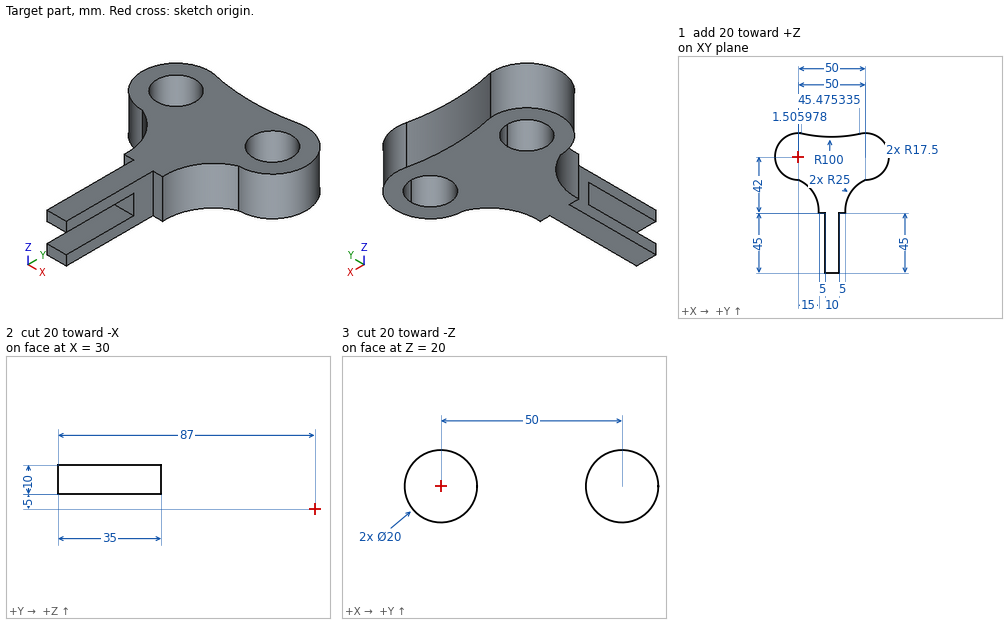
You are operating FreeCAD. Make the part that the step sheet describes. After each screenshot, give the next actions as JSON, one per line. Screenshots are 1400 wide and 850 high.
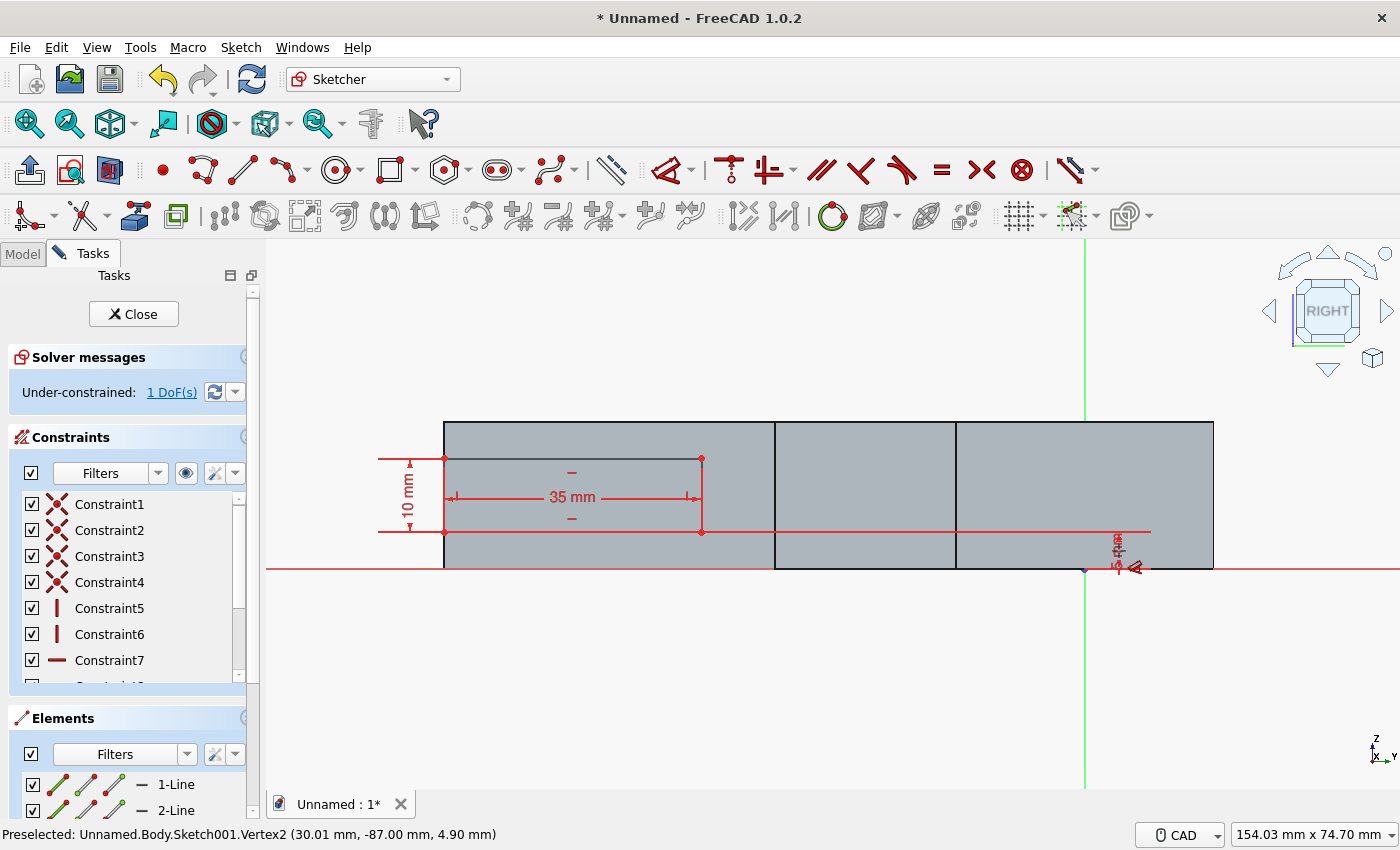
{"action": "left_click", "coordinate": [444, 459]}
{"action": "left_click", "coordinate": [764, 603]}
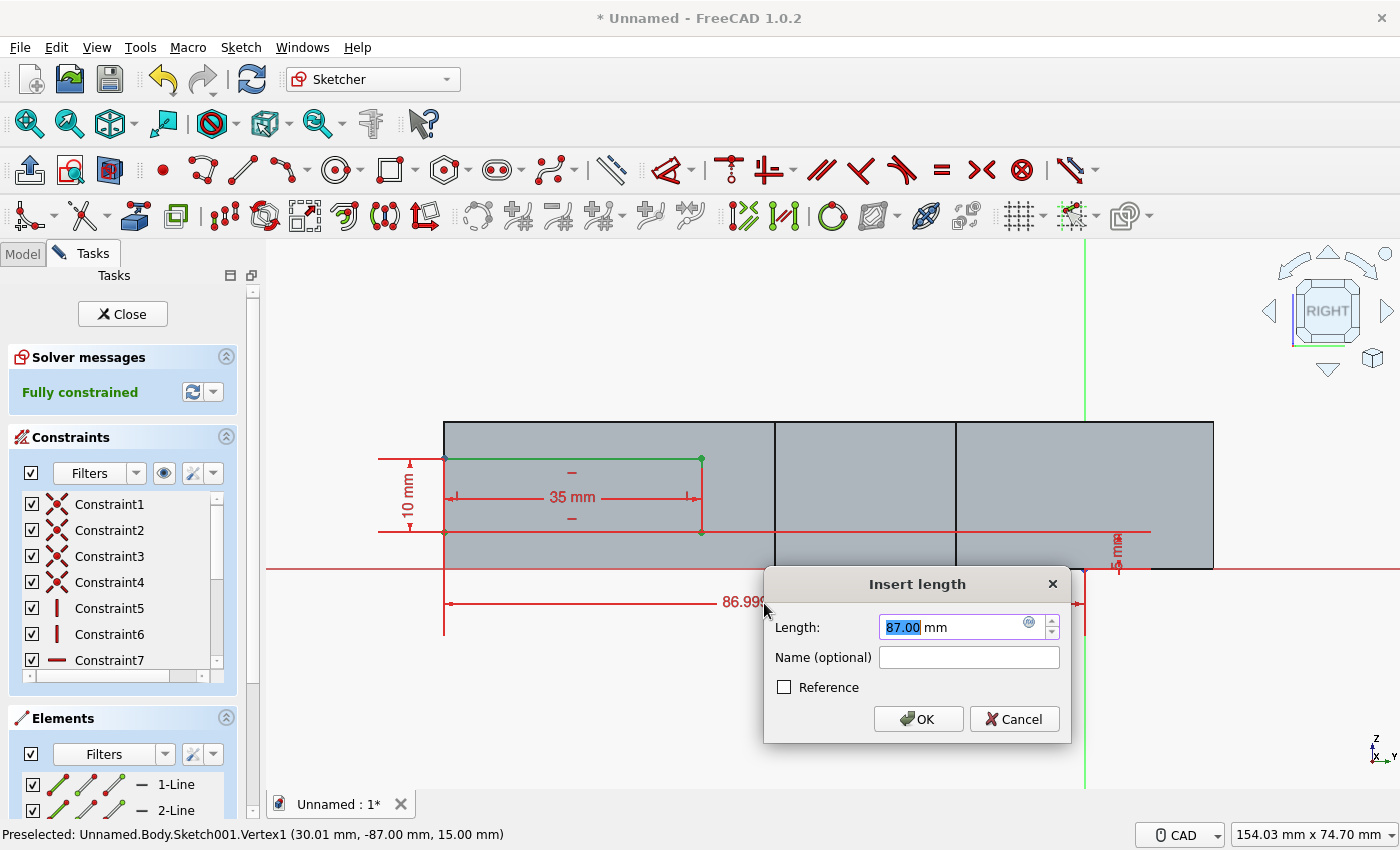
{"action": "type", "text": "87"}
{"action": "key", "text": "Return"}
{"action": "key", "text": "Escape"}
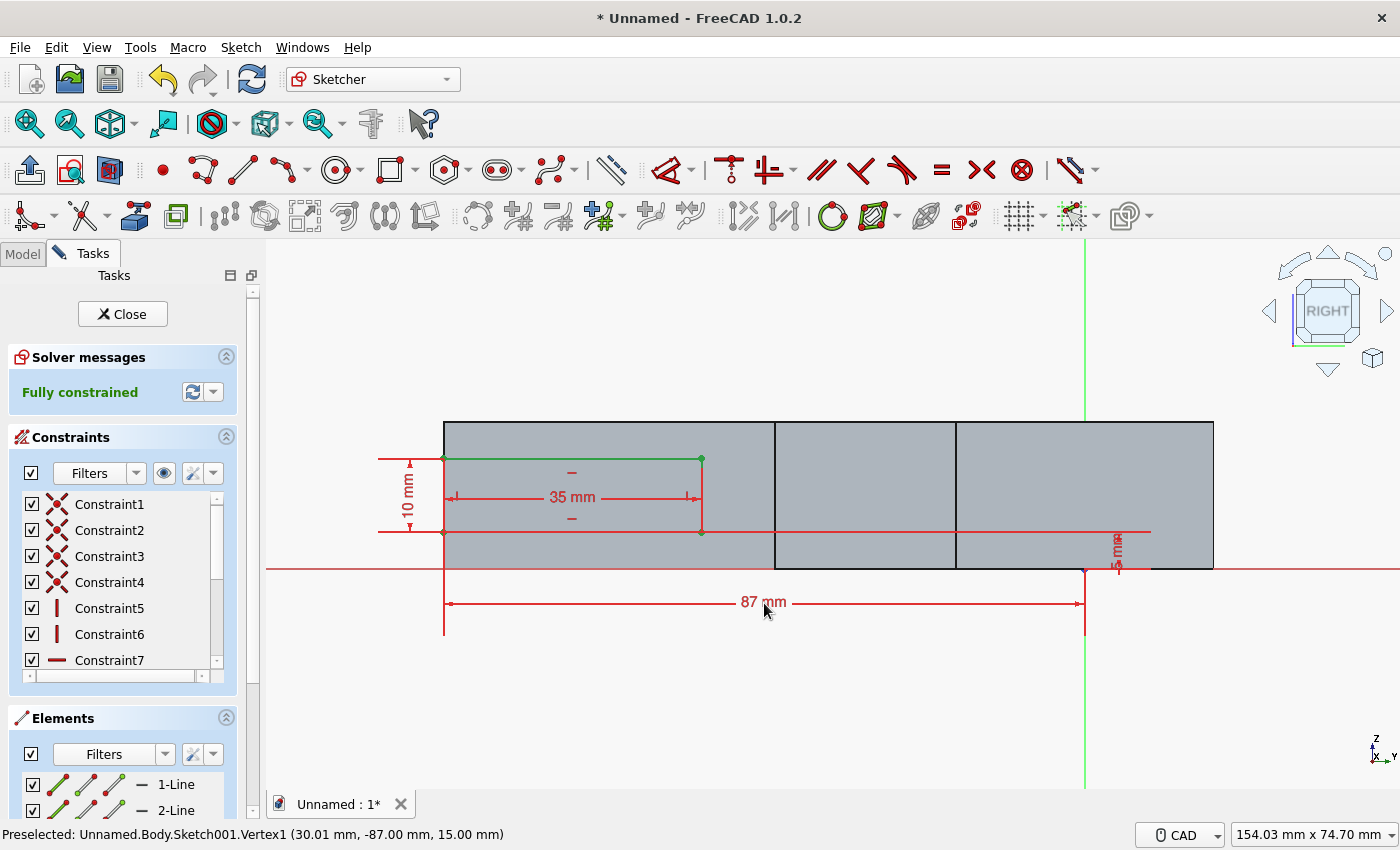
{"action": "left_click", "coordinate": [123, 314]}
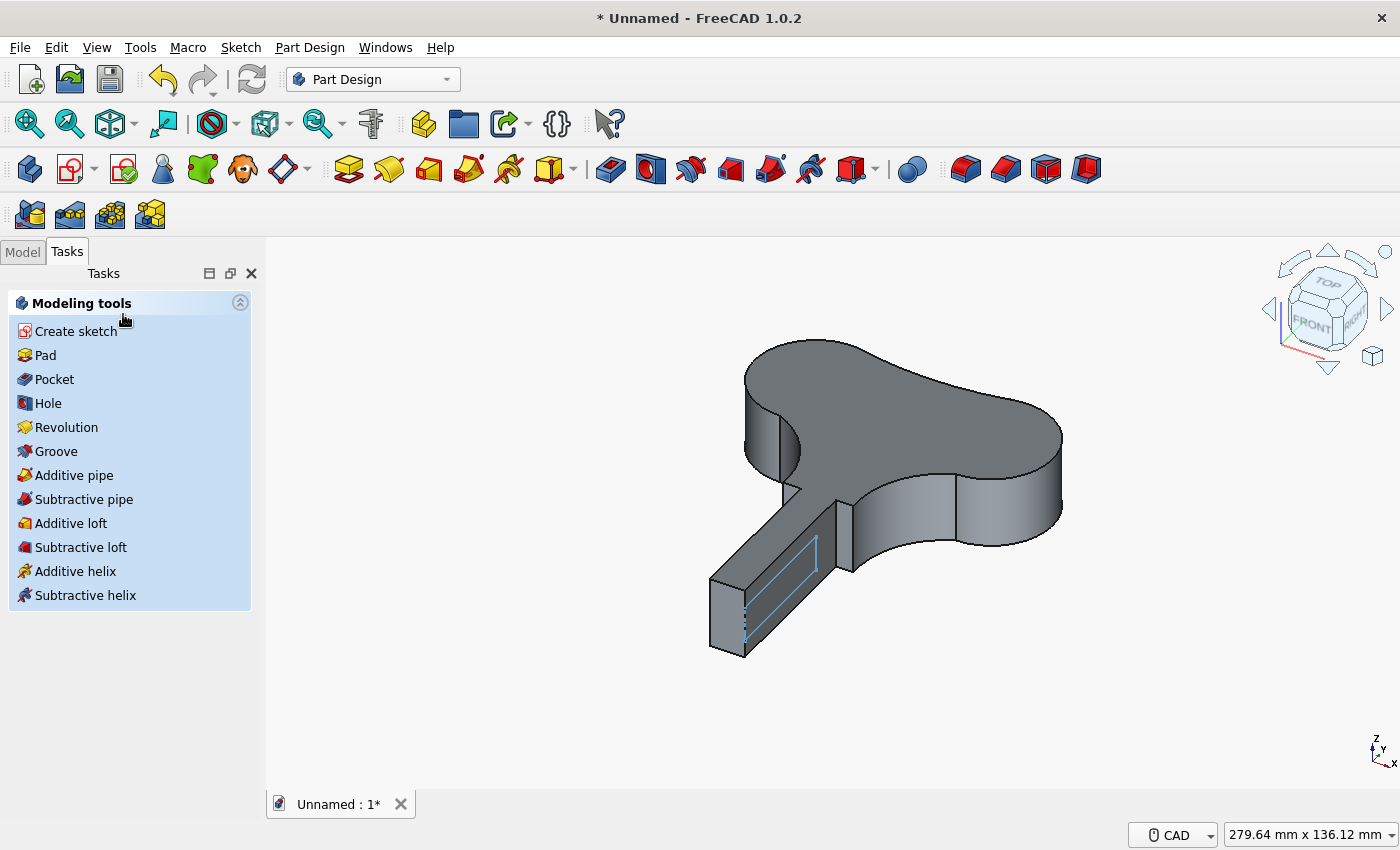
{"action": "left_click", "coordinate": [612, 170]}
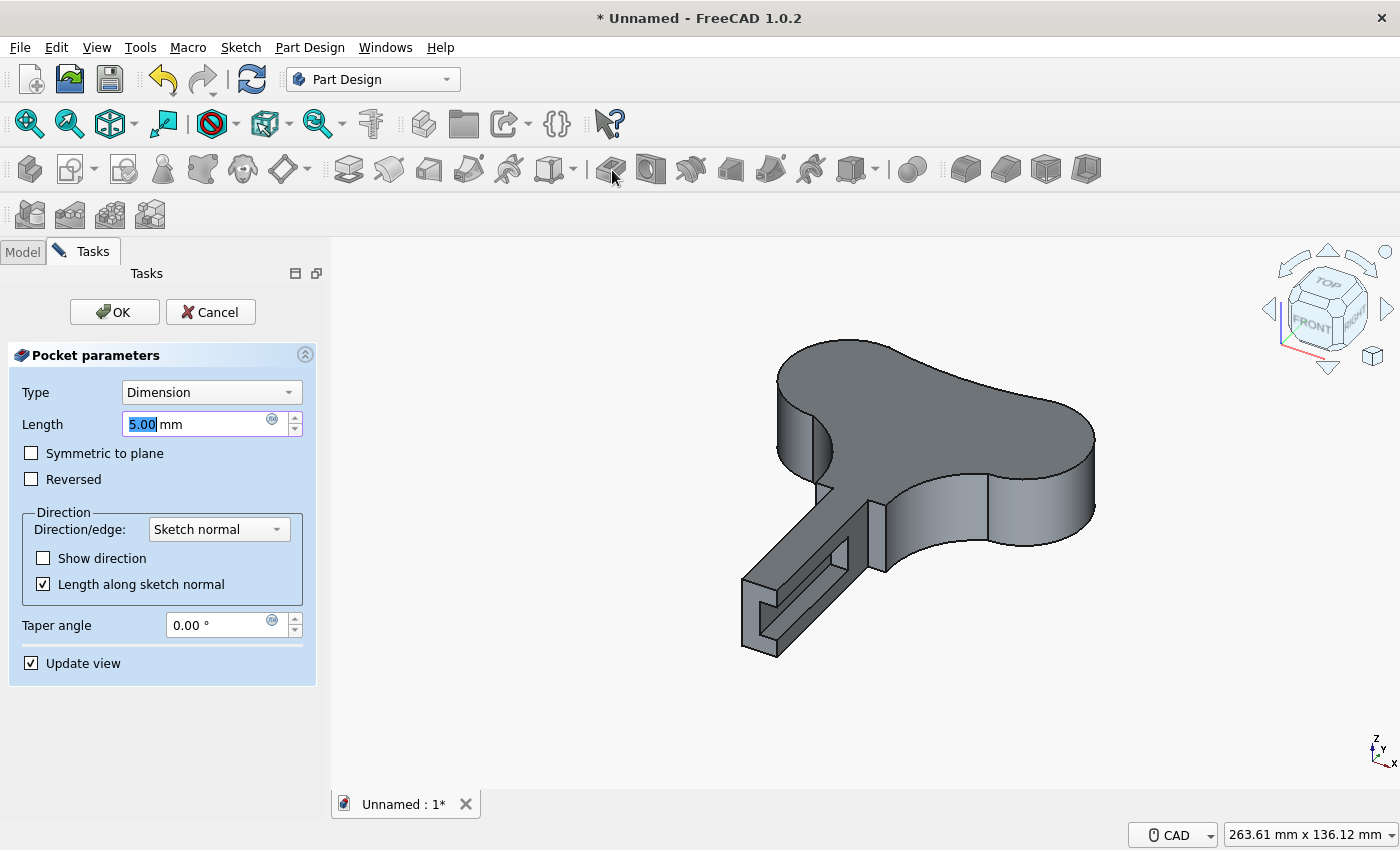
{"action": "type", "text": "20"}
{"action": "key", "text": "Tab"}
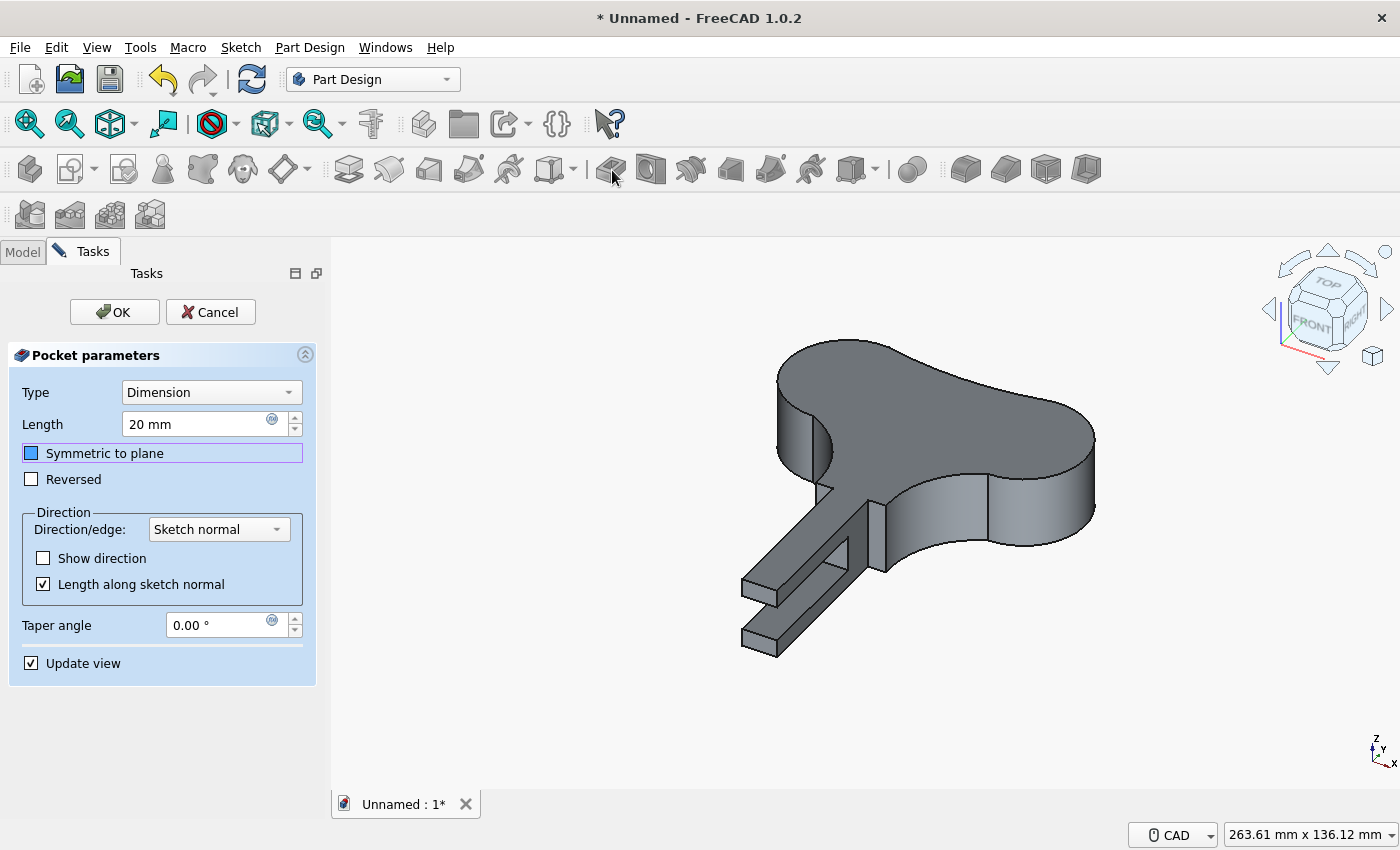
{"action": "left_click", "coordinate": [115, 312]}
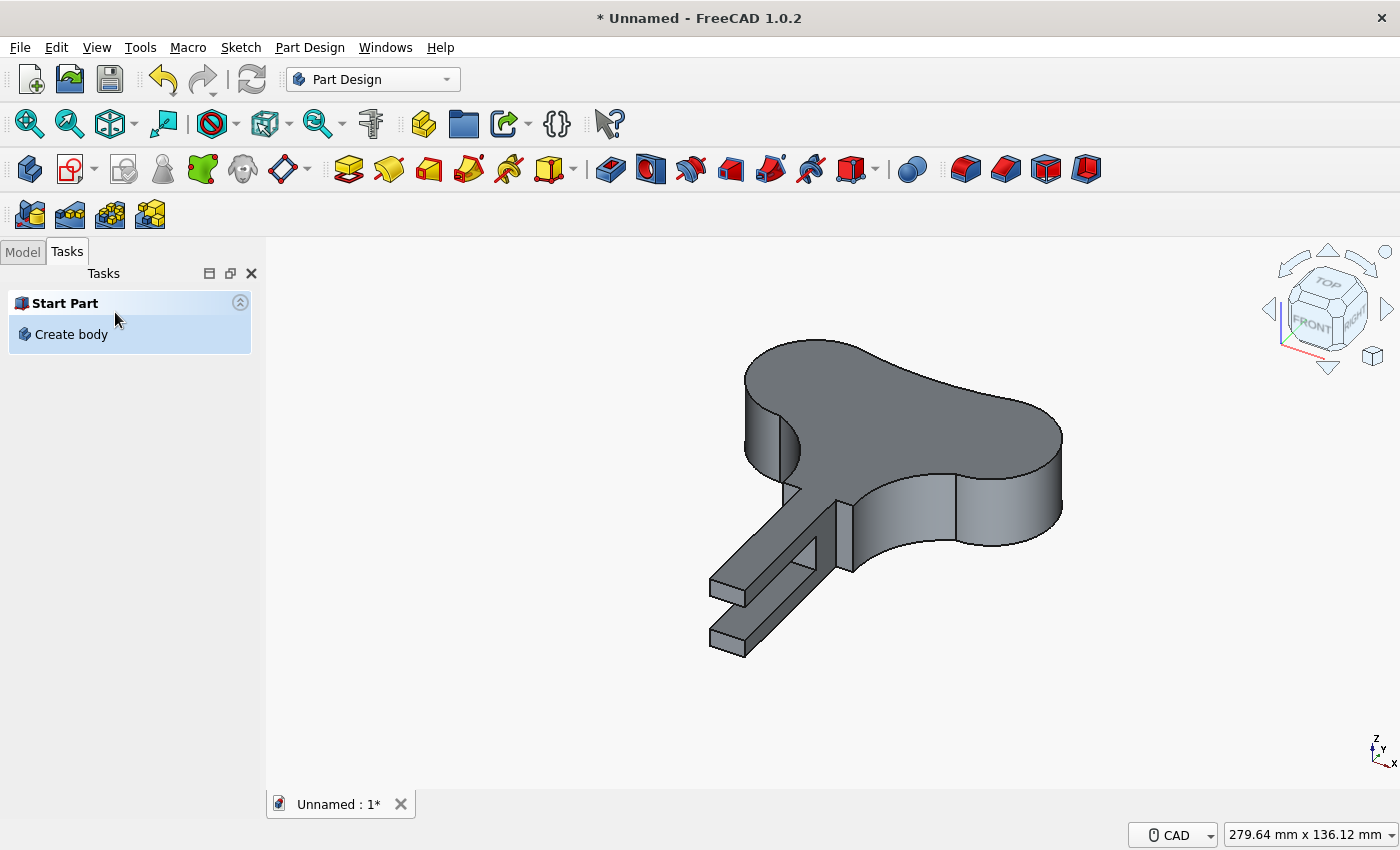
{"action": "left_click", "coordinate": [894, 419]}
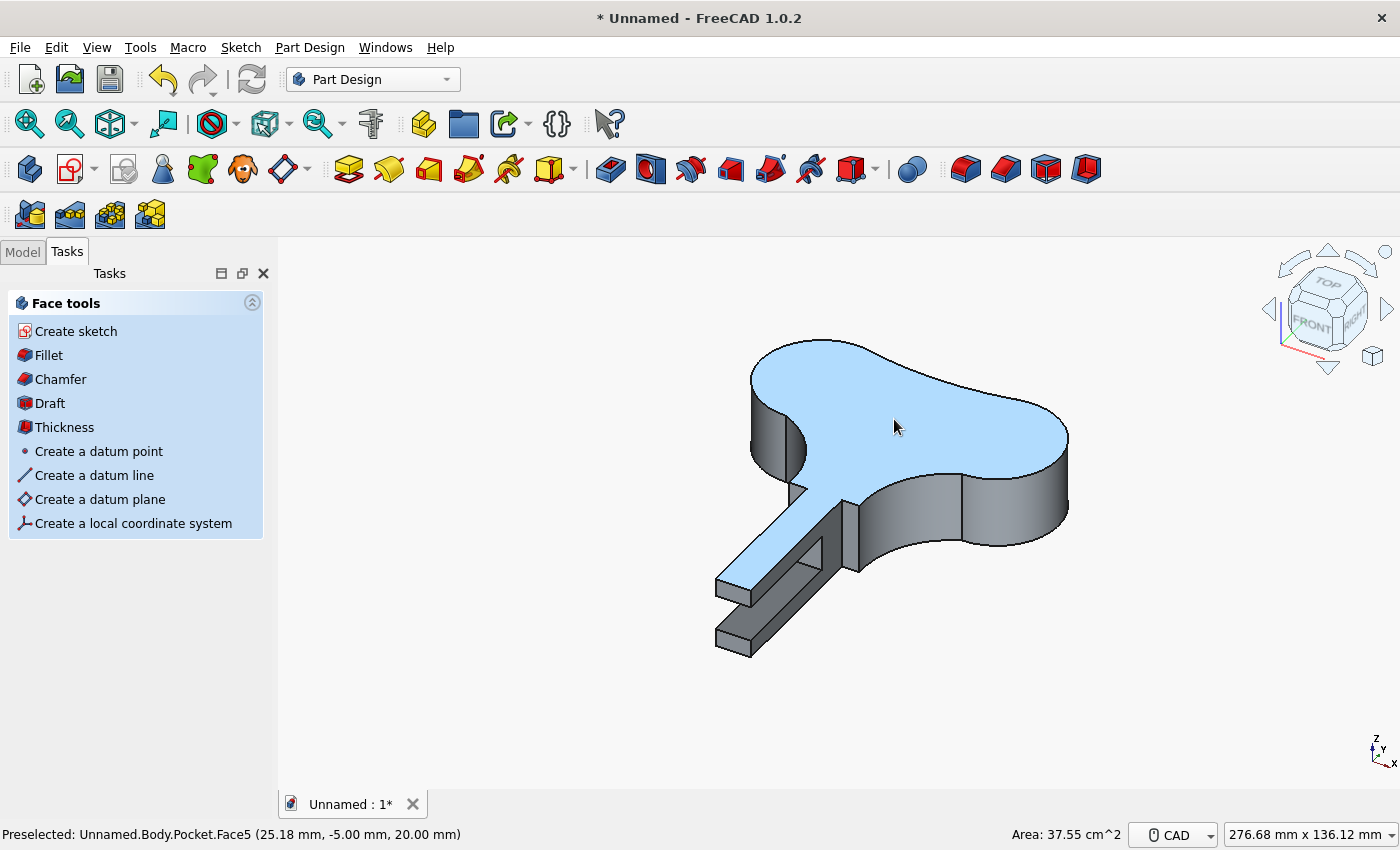
{"action": "left_click", "coordinate": [70, 170]}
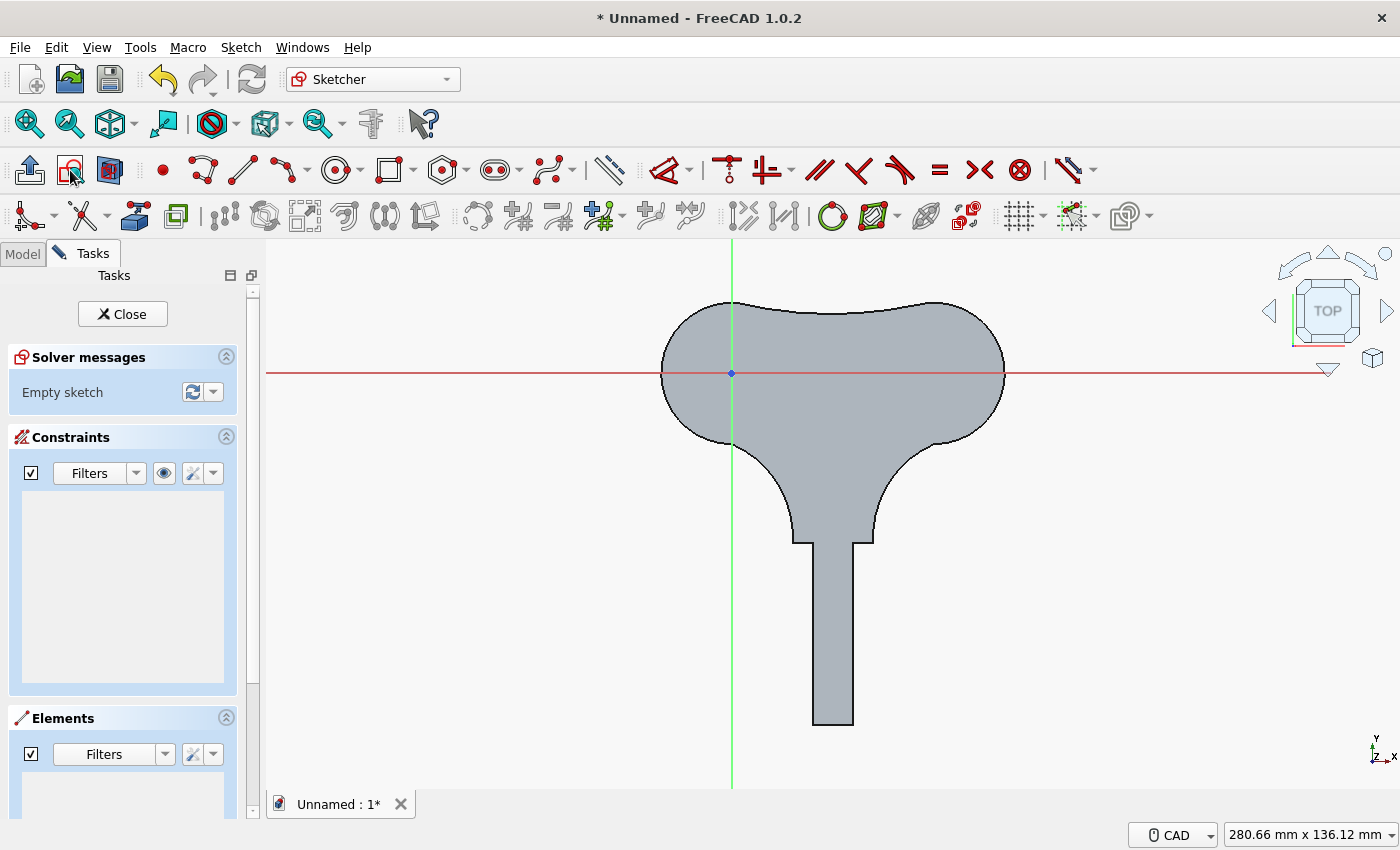
{"action": "scroll", "coordinate": [889, 267], "scroll_direction": "up", "scroll_amount": 4}